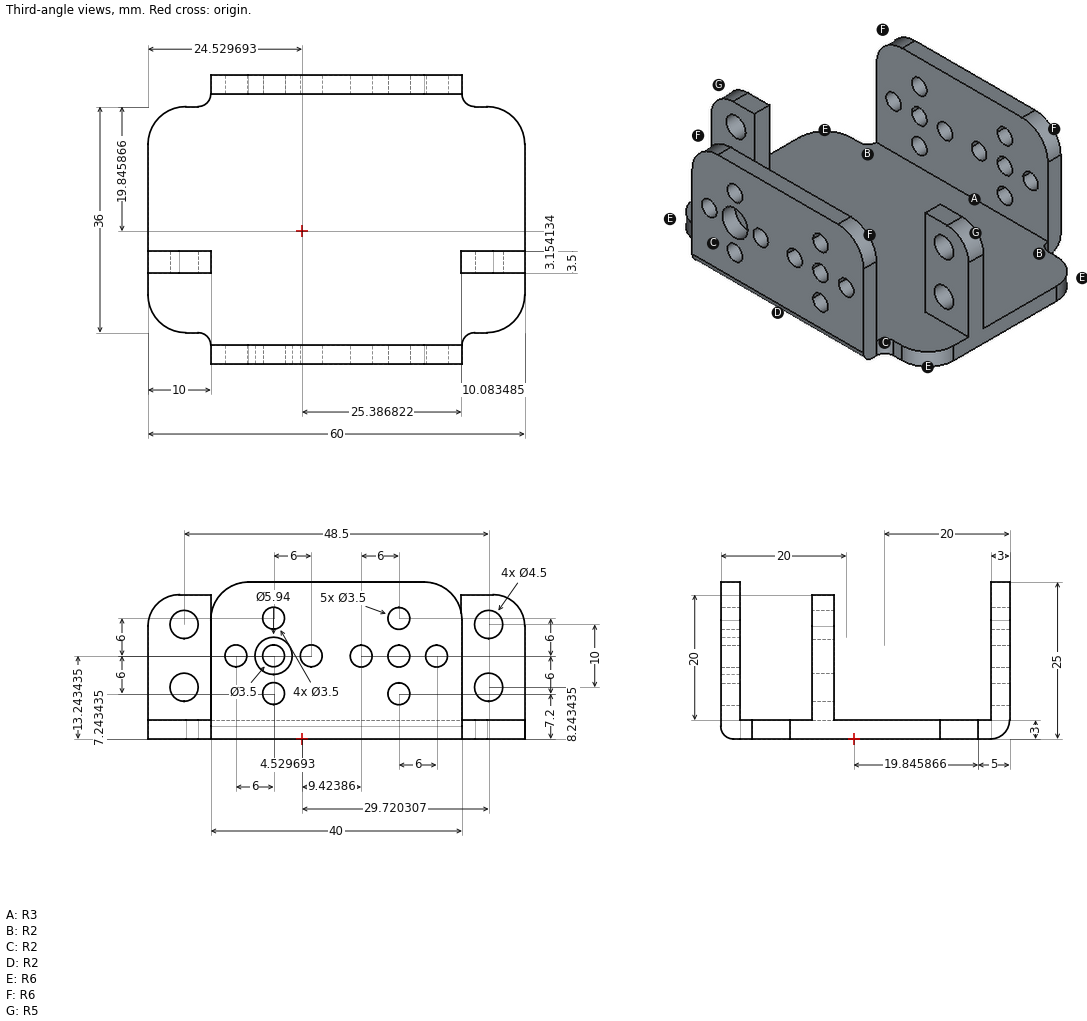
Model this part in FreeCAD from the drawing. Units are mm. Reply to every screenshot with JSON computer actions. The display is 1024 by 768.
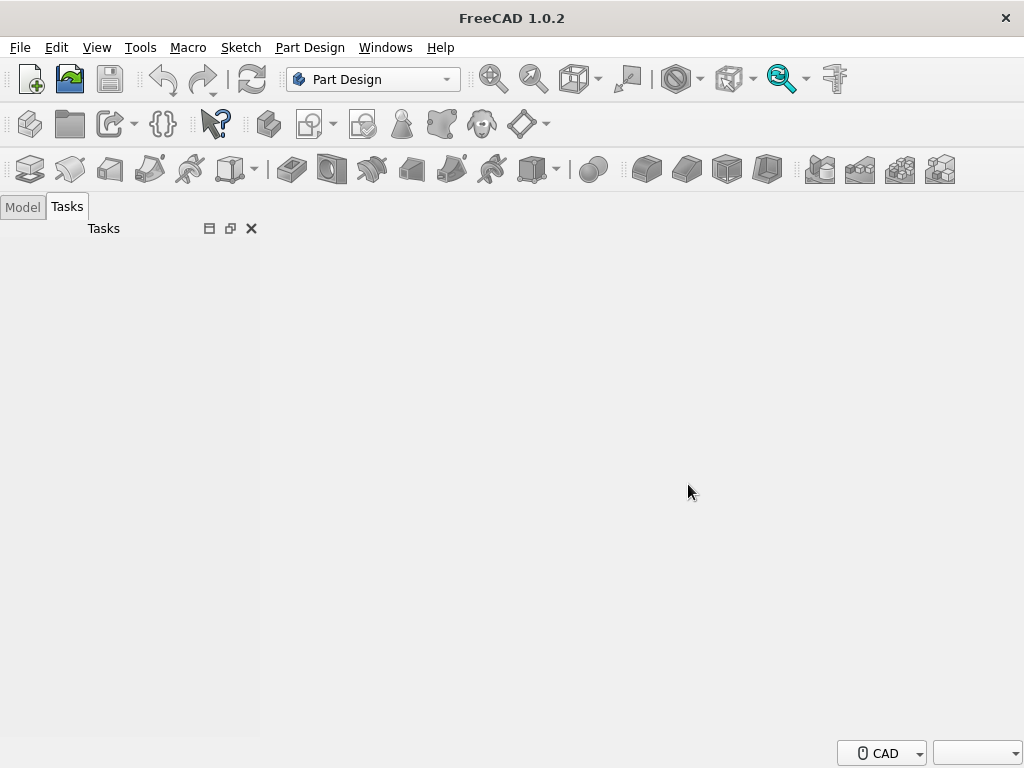
{"action": "left_click", "coordinate": [30, 80]}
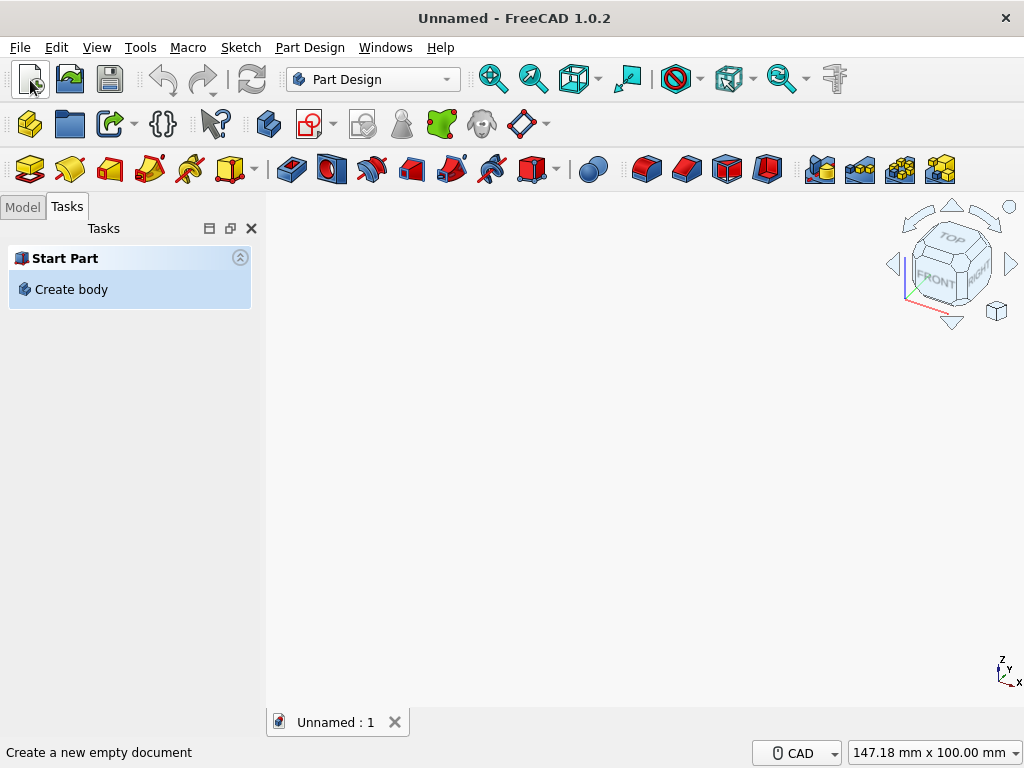
{"action": "left_click", "coordinate": [310, 124]}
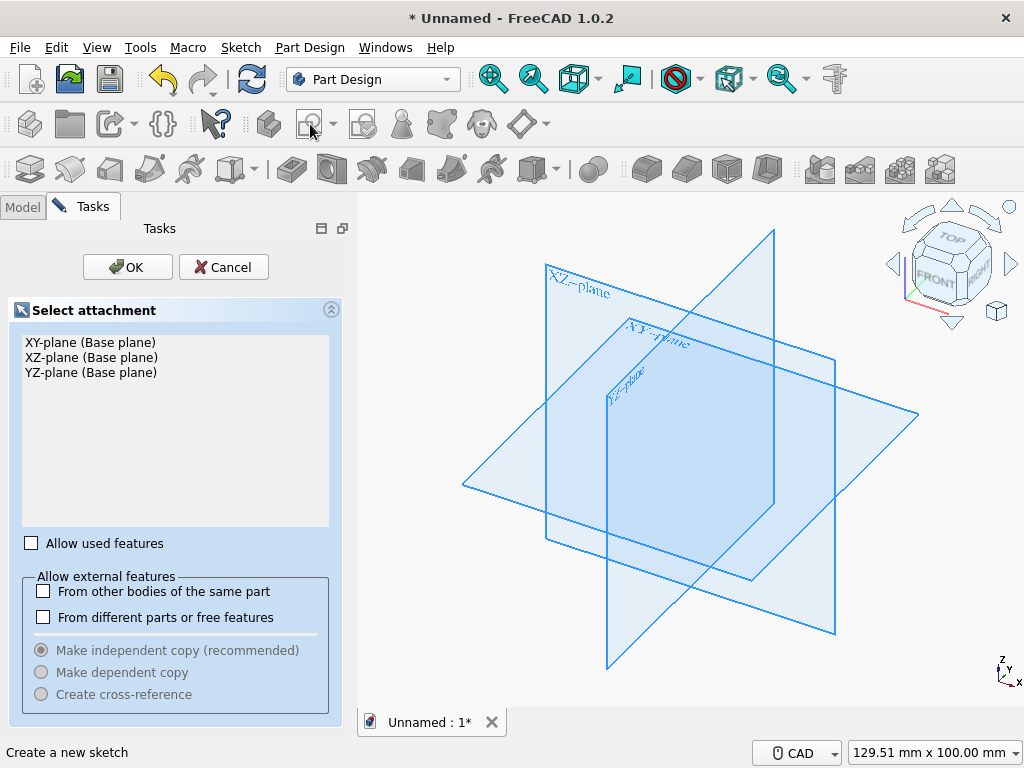
{"action": "left_click", "coordinate": [82, 342]}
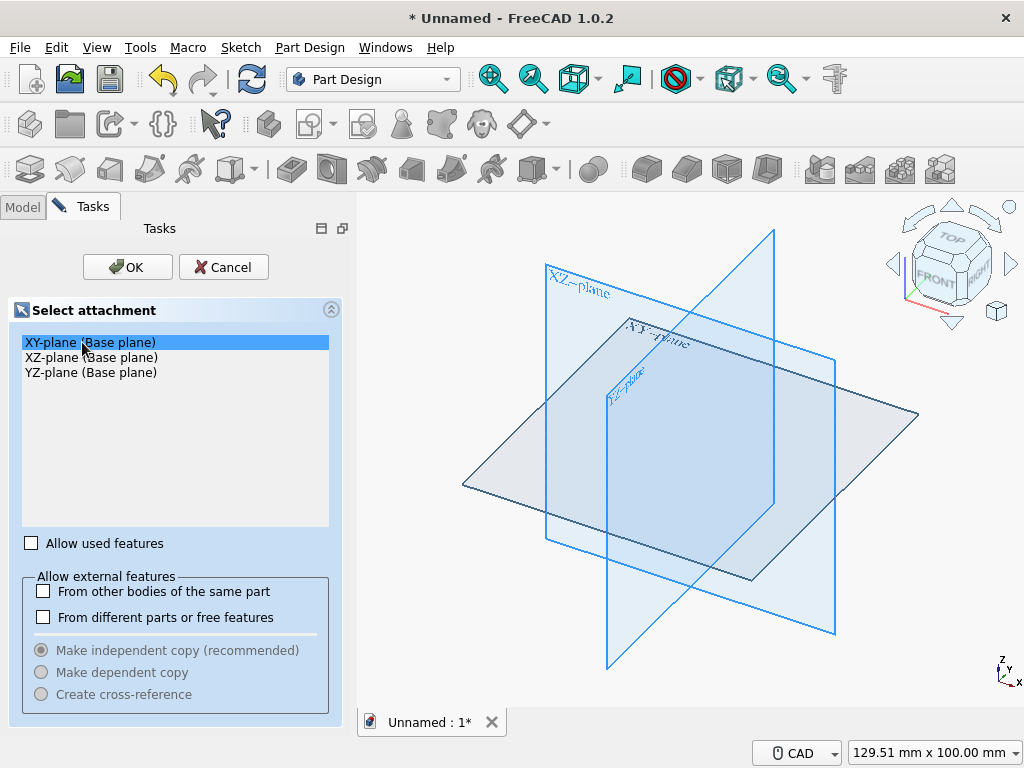
{"action": "left_click", "coordinate": [128, 267]}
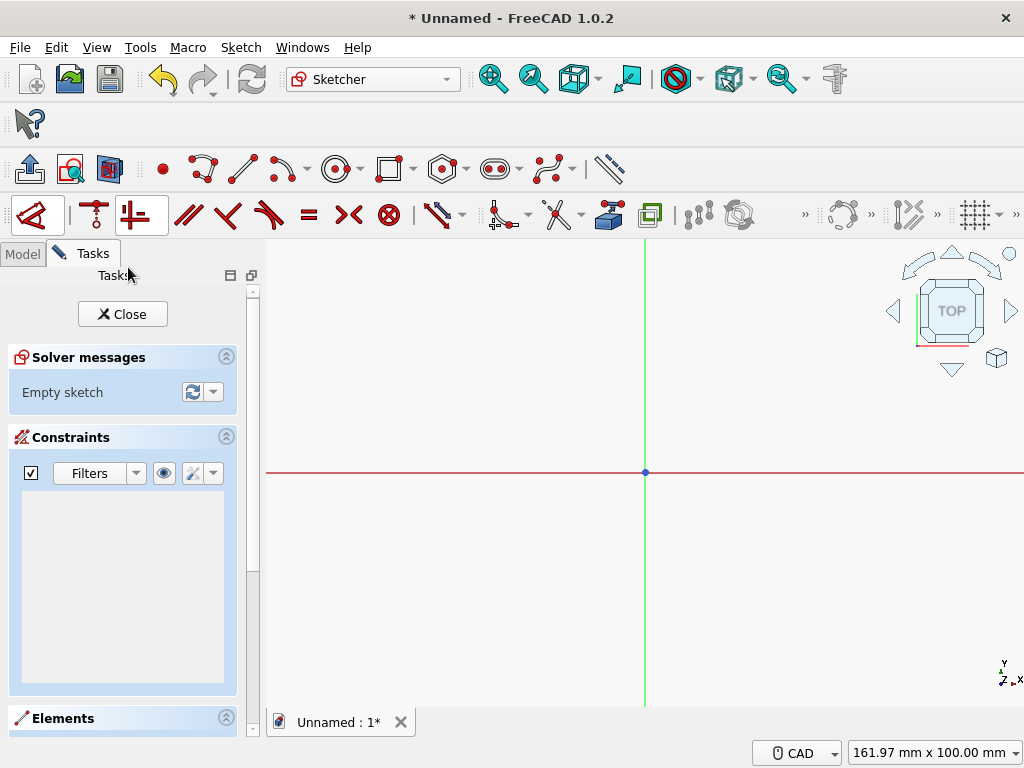
{"action": "scroll", "coordinate": [859, 447], "scroll_direction": "up", "scroll_amount": 2}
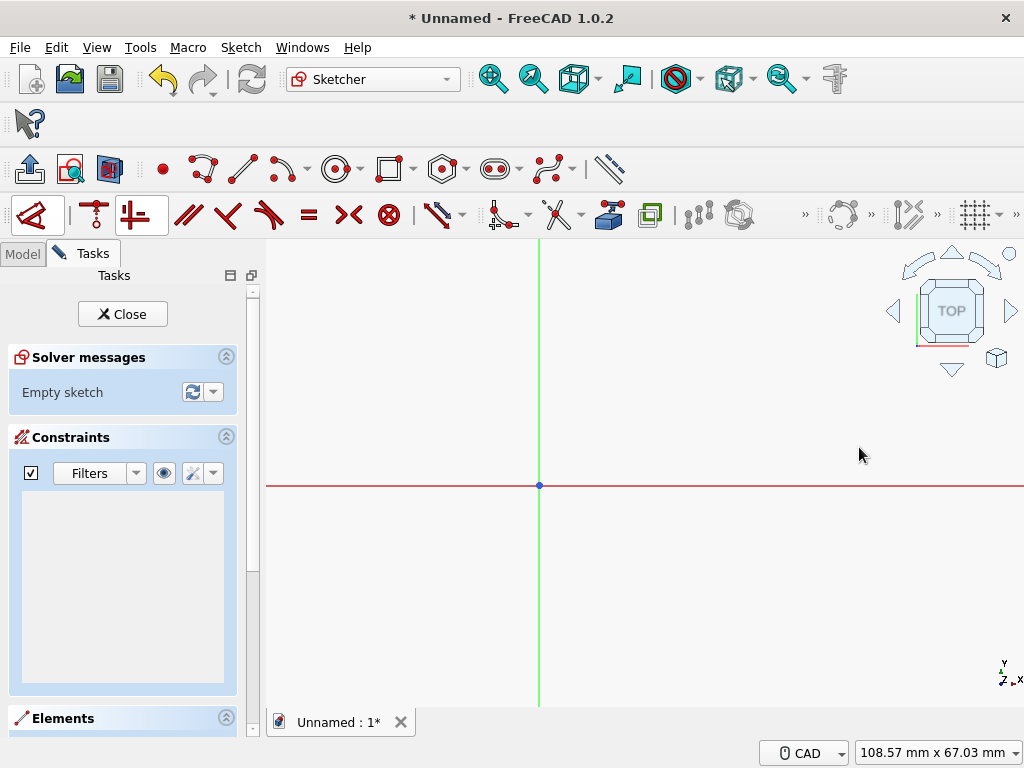
{"action": "left_click", "coordinate": [390, 170]}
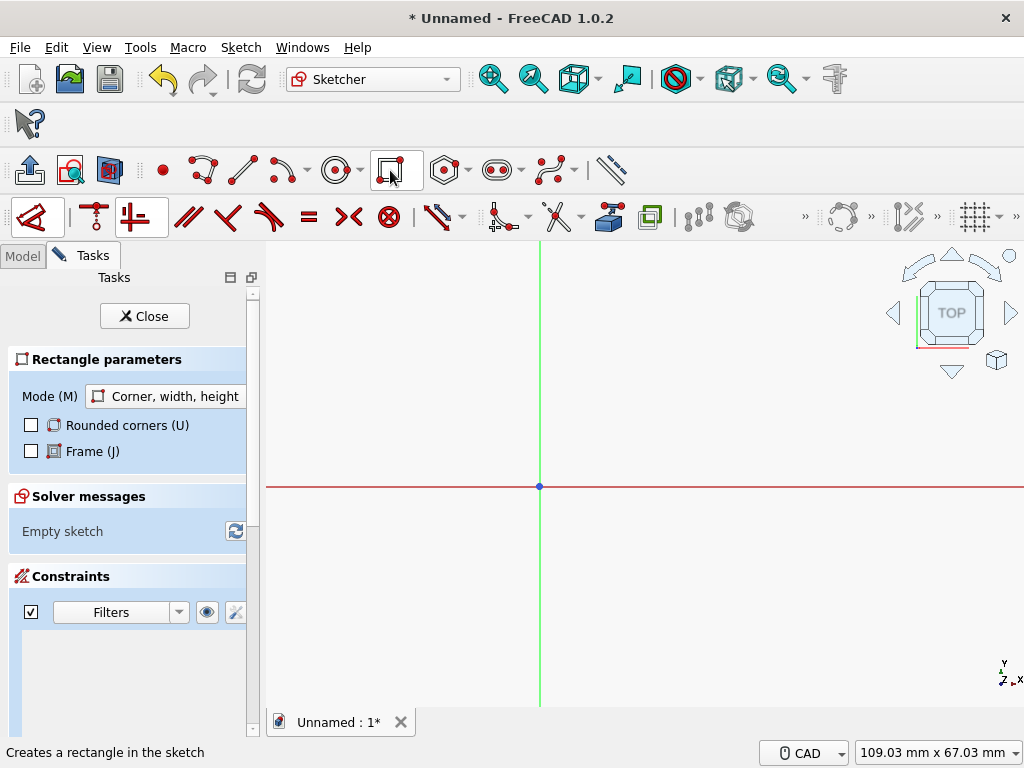
{"action": "left_click", "coordinate": [369, 349]}
{"action": "left_click", "coordinate": [786, 599]}
{"action": "key", "text": "Escape"}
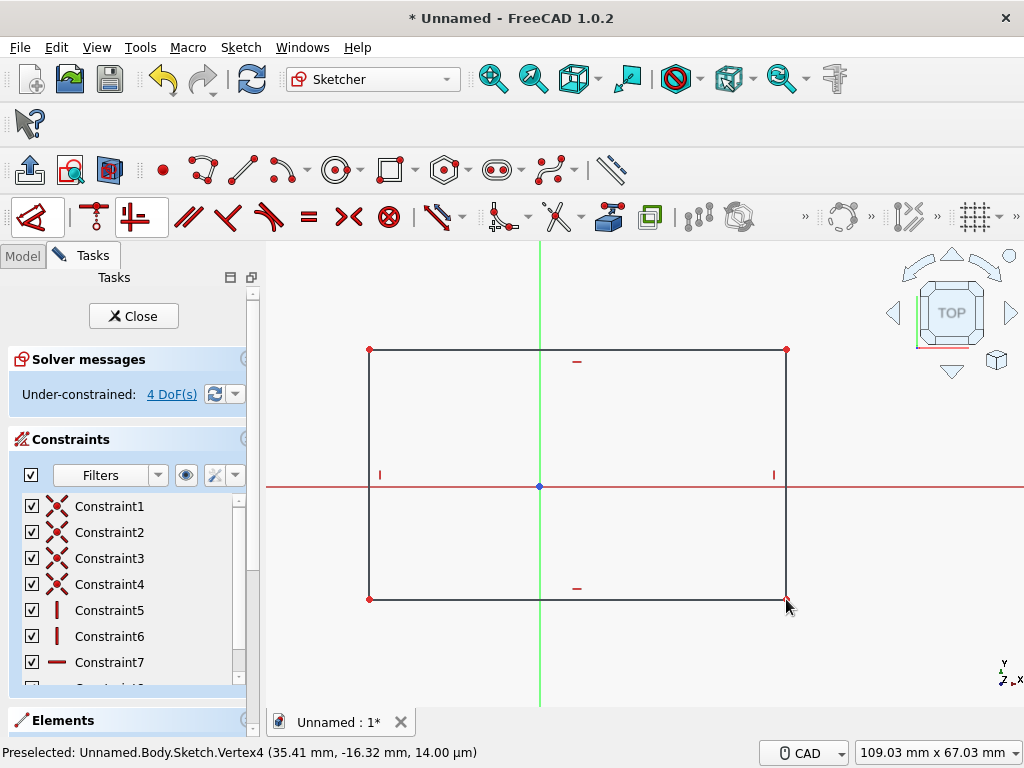
{"action": "left_click", "coordinate": [32, 218]}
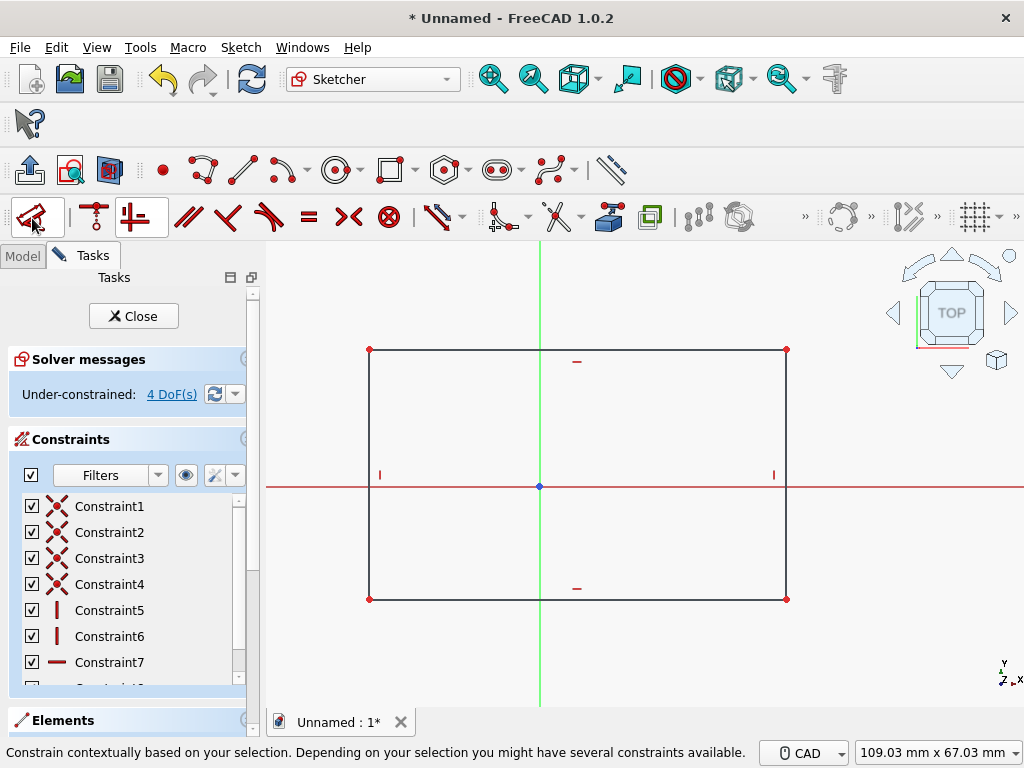
{"action": "left_click", "coordinate": [369, 425]}
{"action": "left_click", "coordinate": [335, 417]}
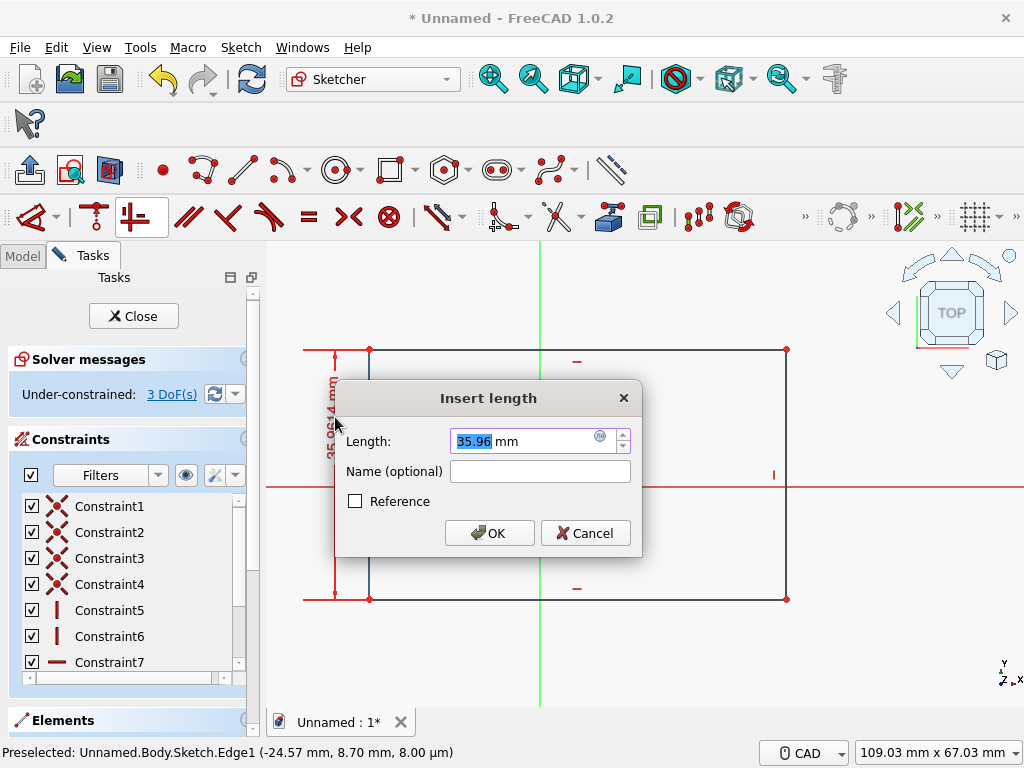
{"action": "type", "text": "36"}
{"action": "key", "text": "Return"}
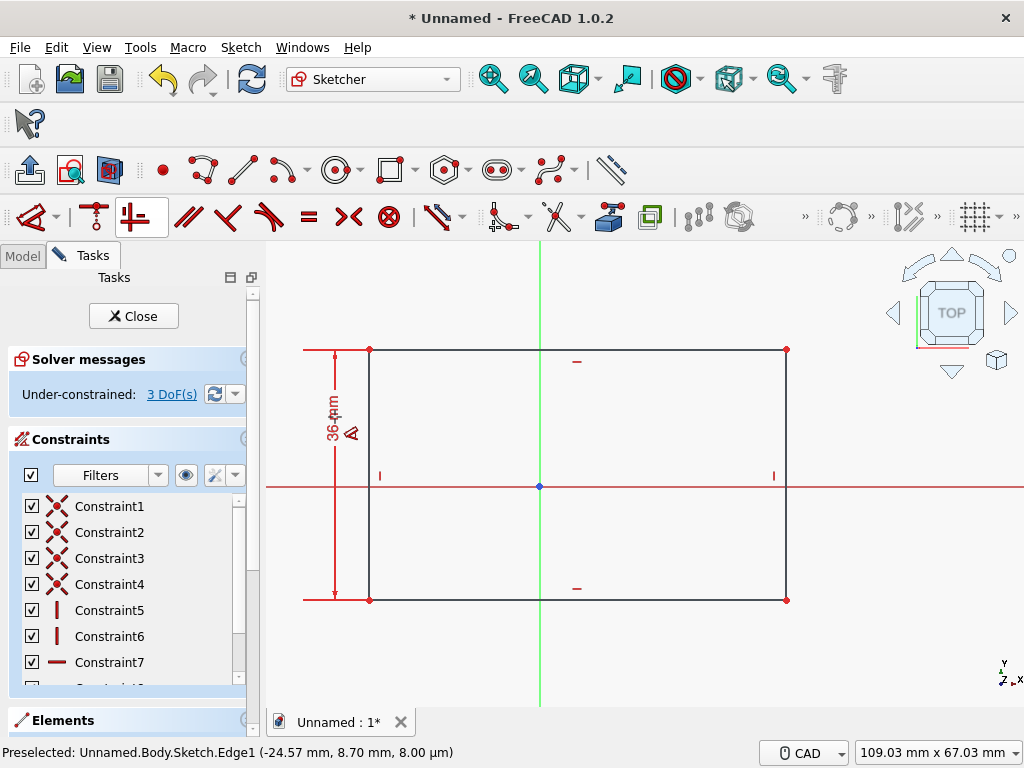
{"action": "left_click", "coordinate": [494, 600]}
{"action": "left_click", "coordinate": [577, 634]}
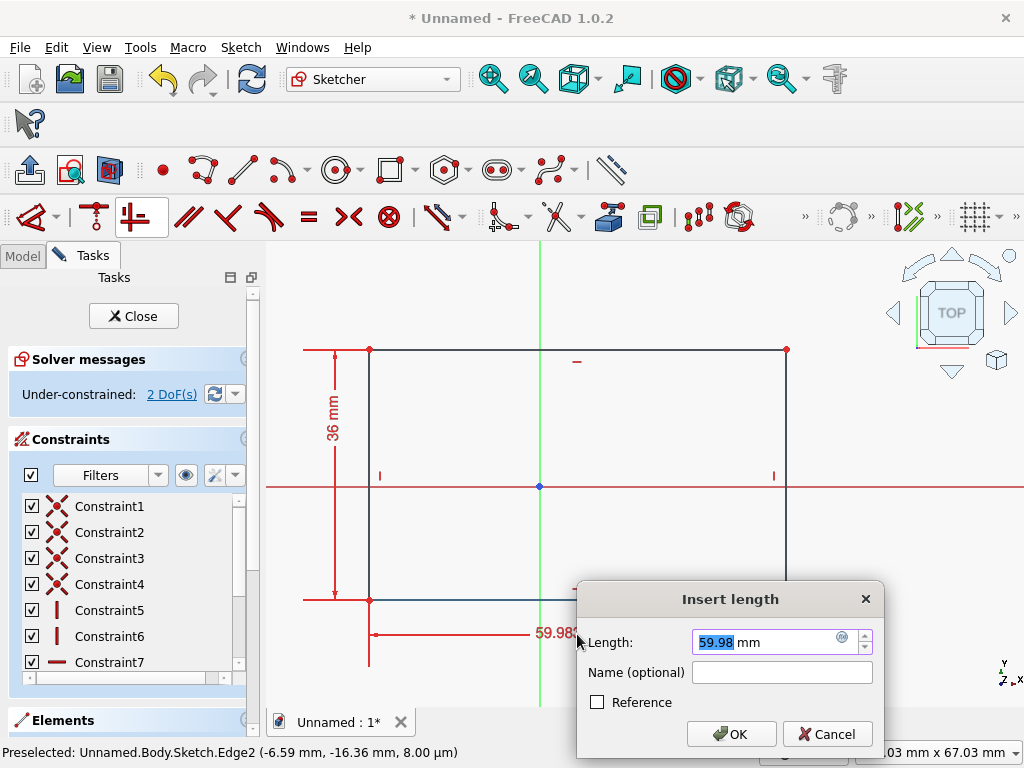
{"action": "type", "text": "60"}
{"action": "key", "text": "Return"}